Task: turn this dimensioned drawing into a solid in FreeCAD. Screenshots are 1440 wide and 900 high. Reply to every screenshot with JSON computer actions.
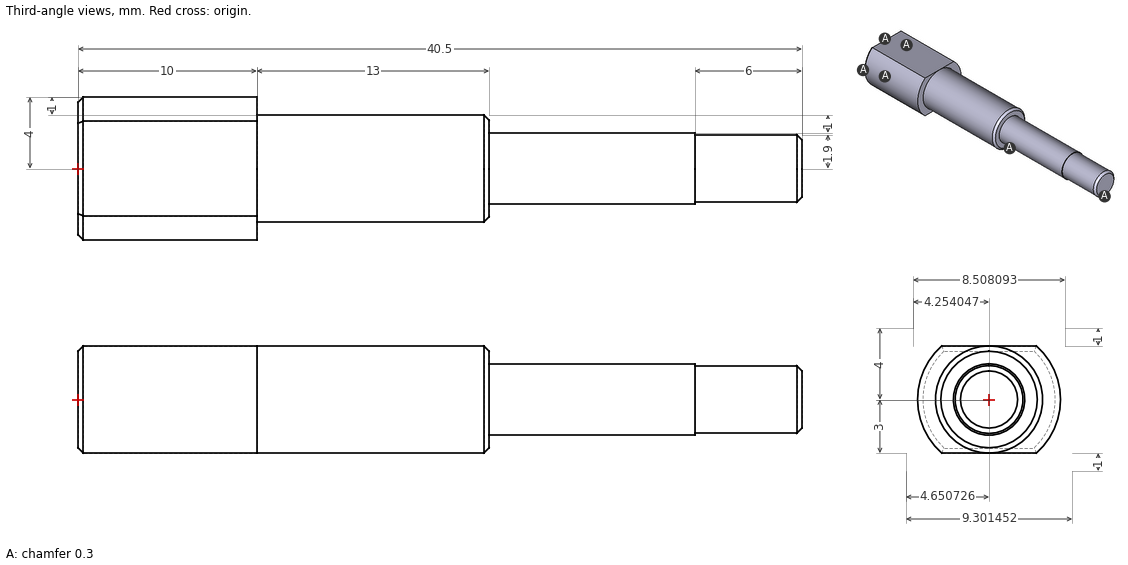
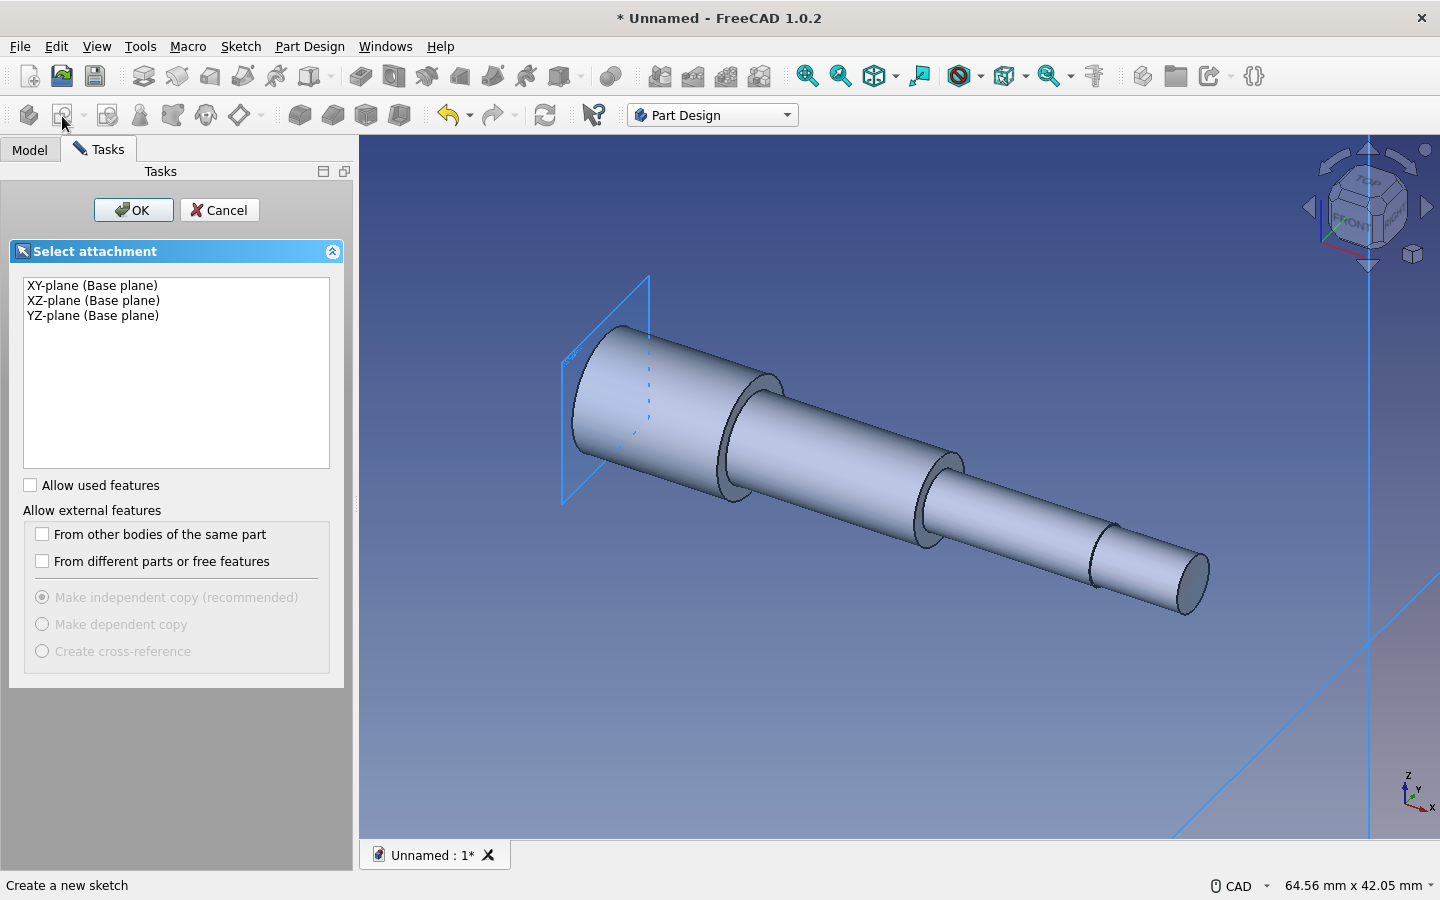
{"action": "left_click", "coordinate": [84, 316]}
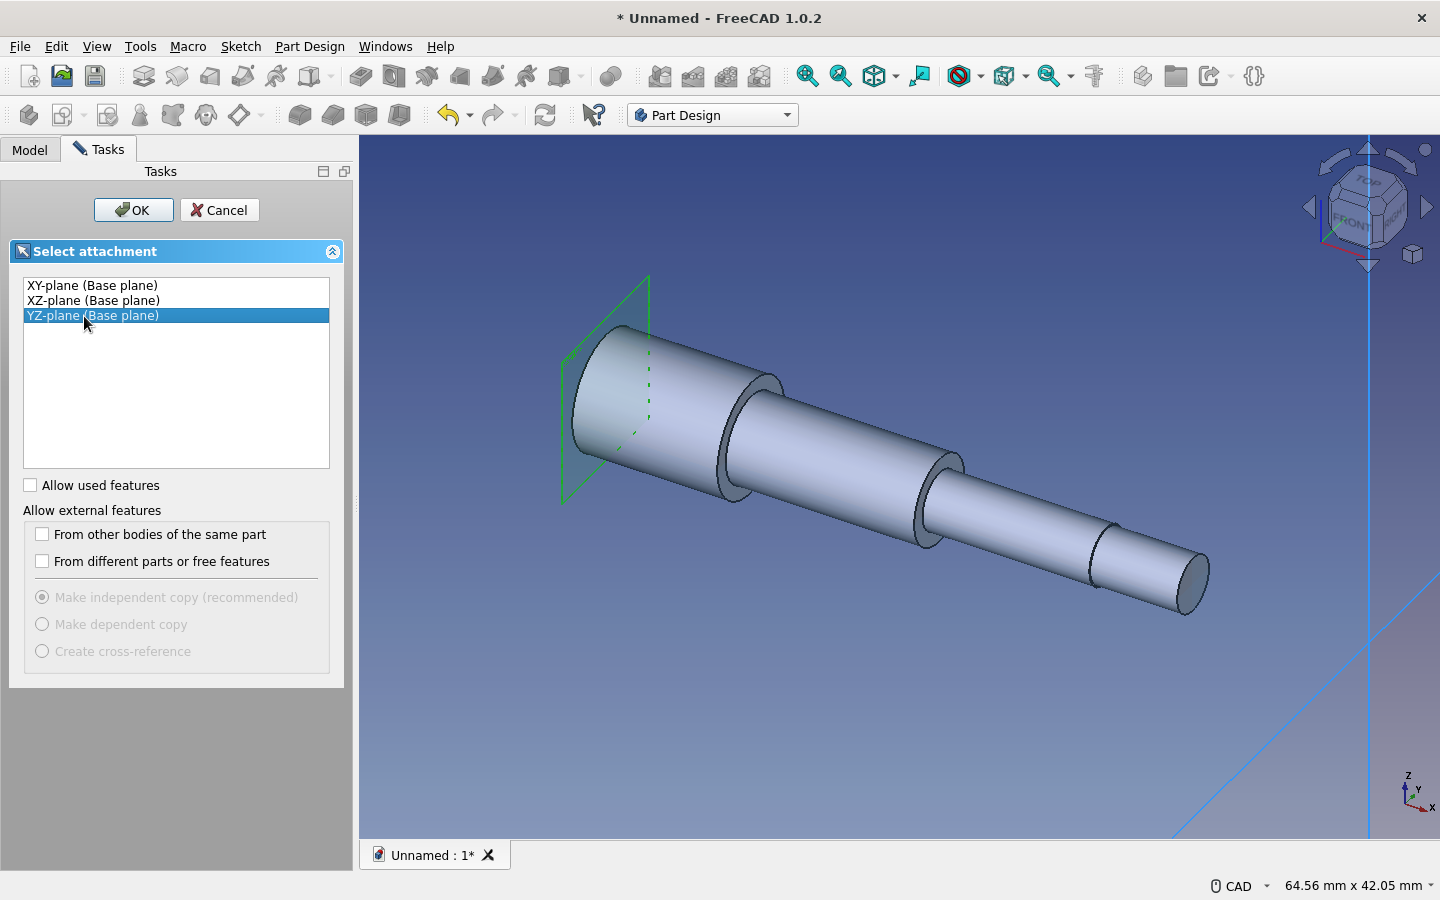
{"action": "left_click", "coordinate": [134, 210]}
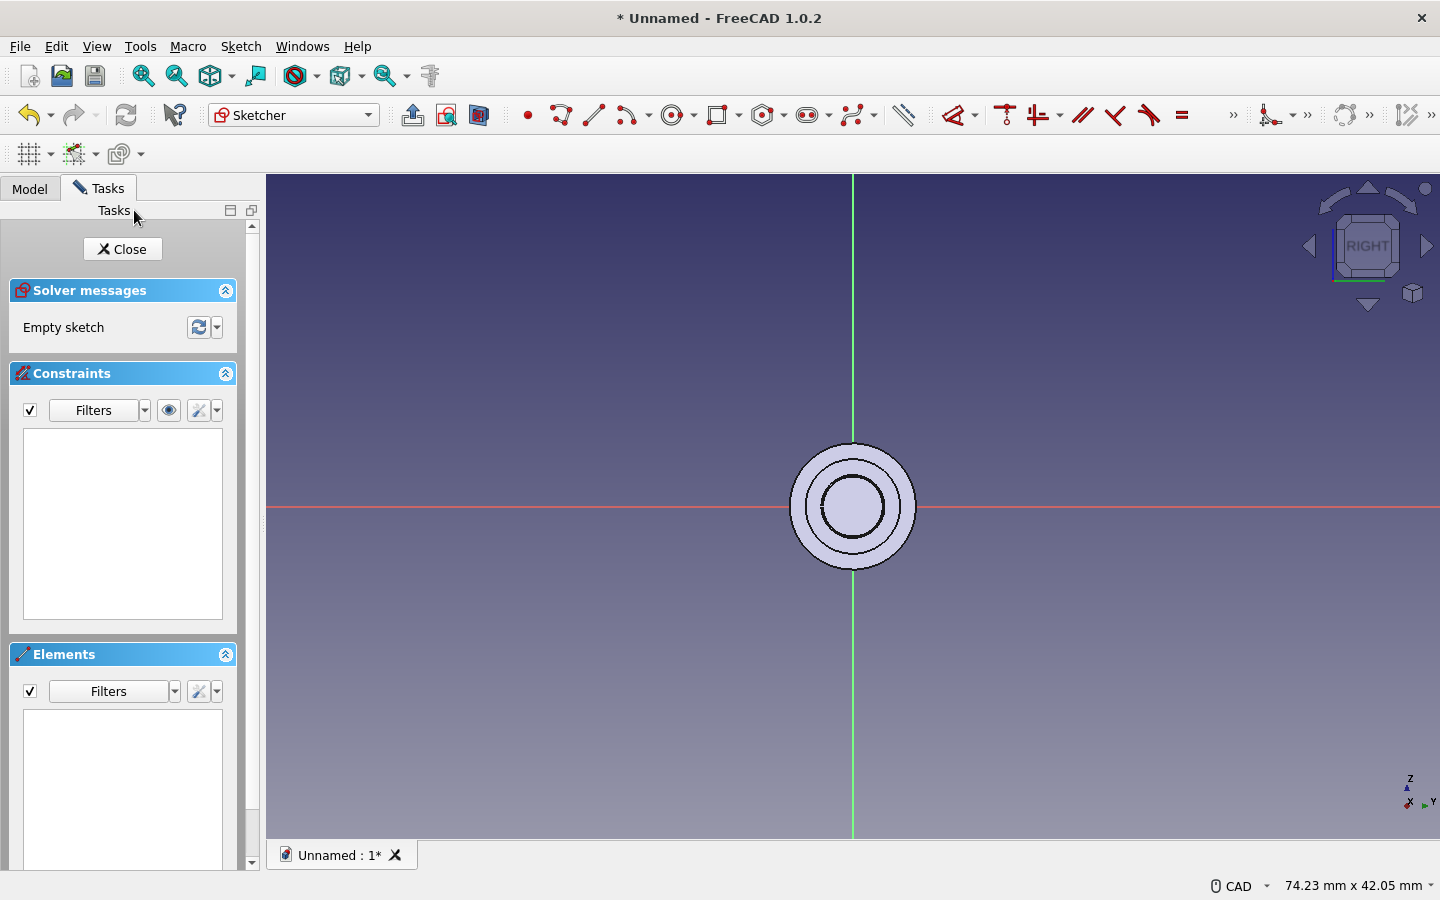
{"action": "left_click", "coordinate": [479, 116]}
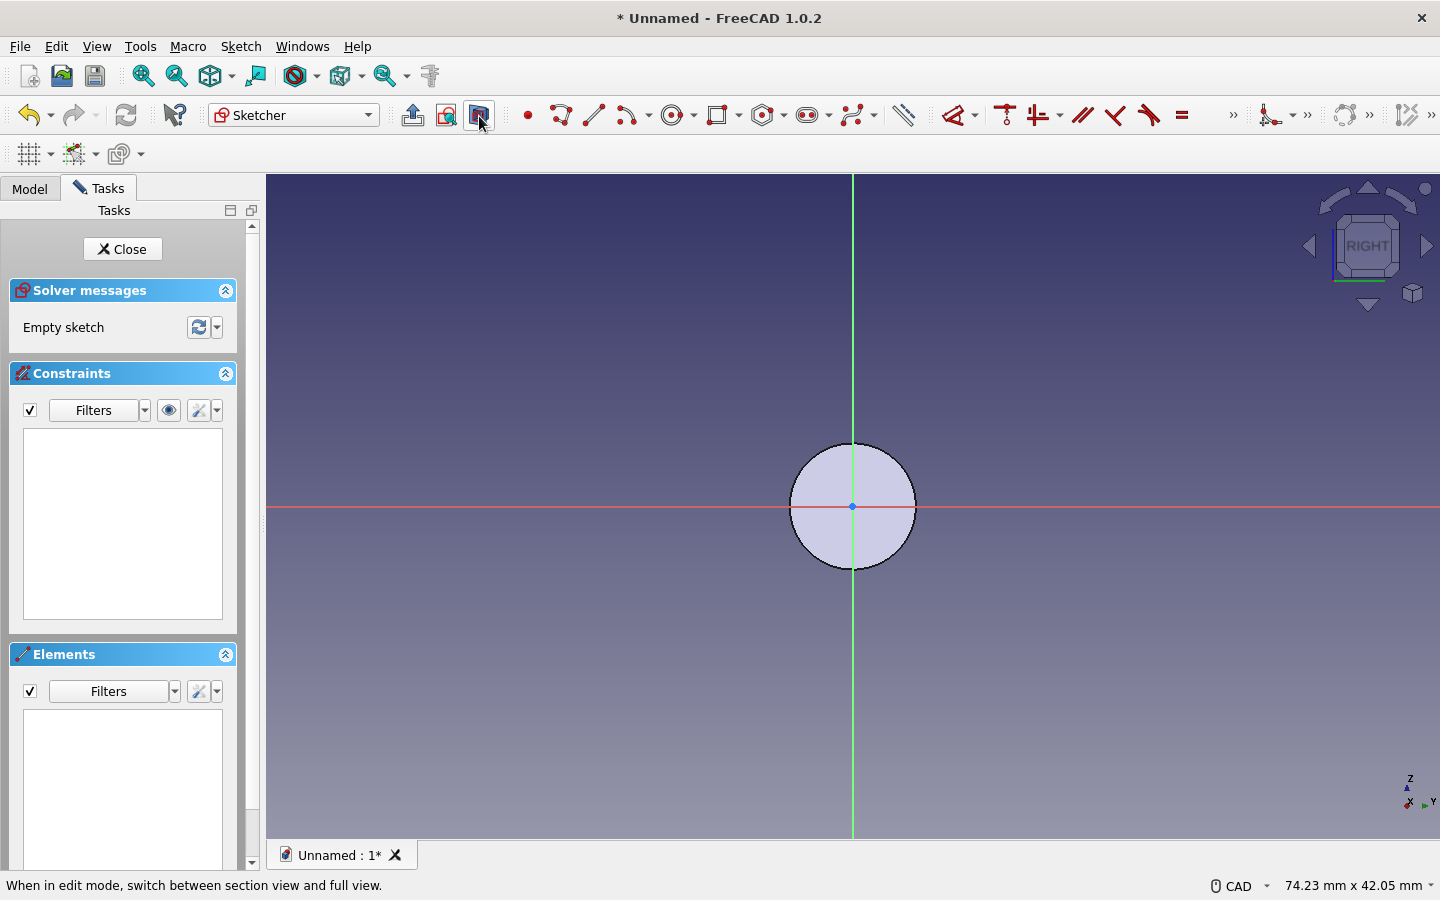
{"action": "scroll", "coordinate": [870, 546], "scroll_direction": "up", "scroll_amount": 8}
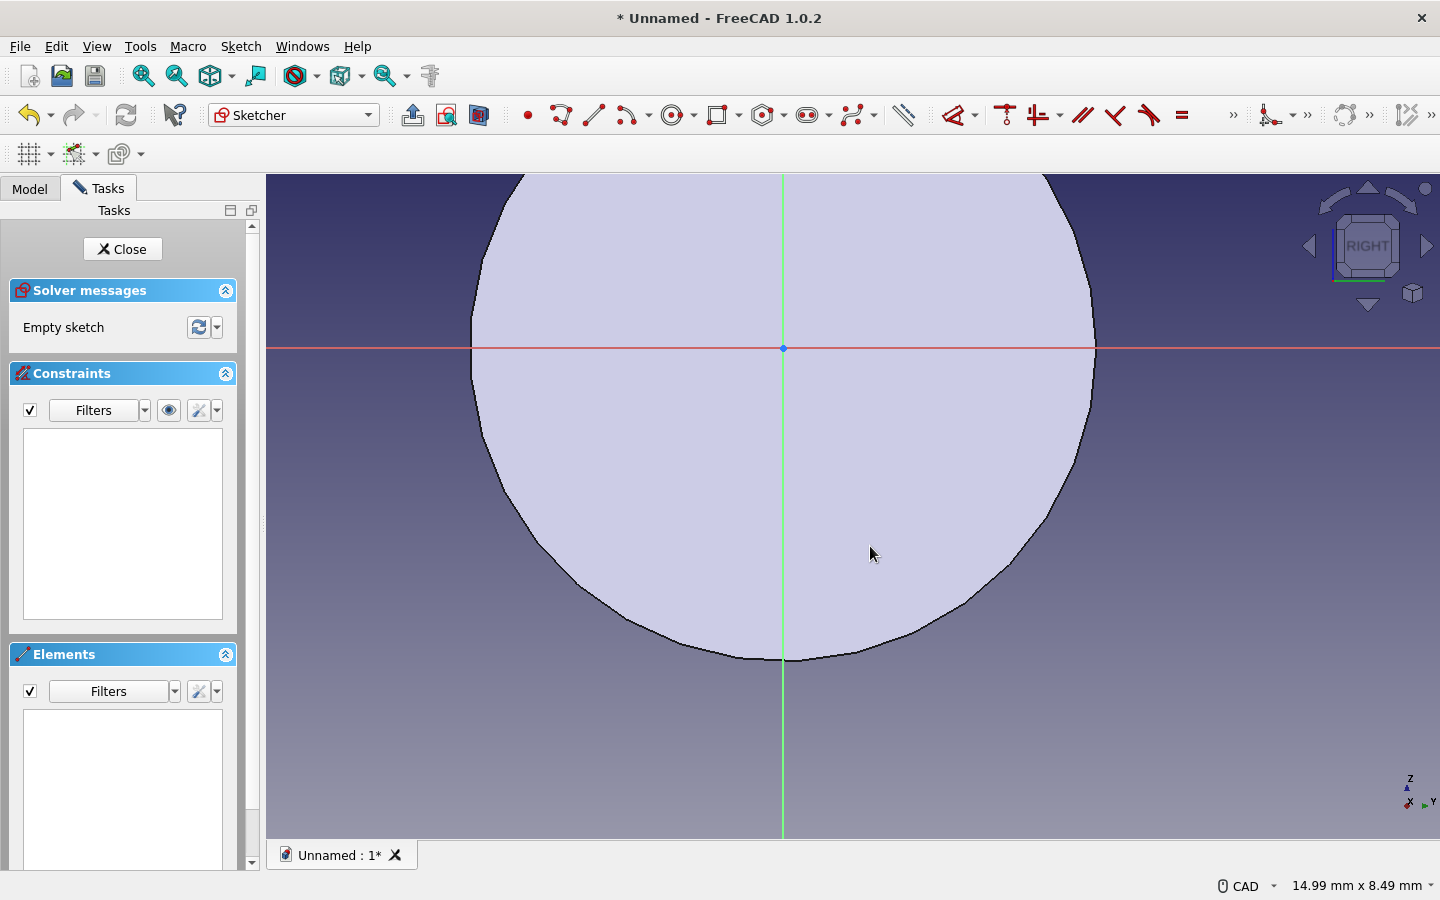
{"action": "left_click", "coordinate": [716, 116]}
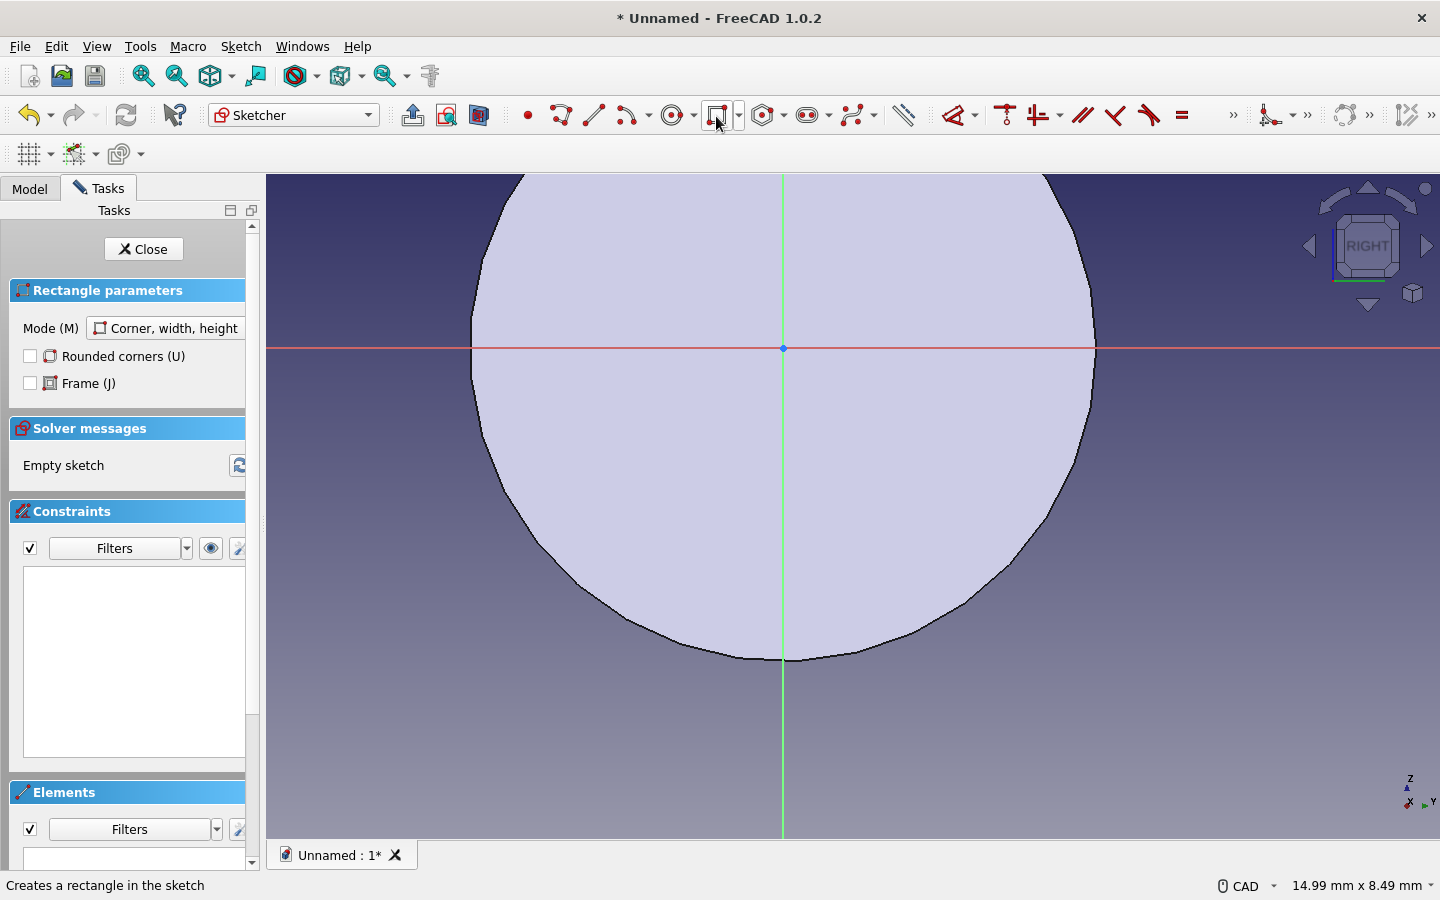
{"action": "left_click", "coordinate": [419, 583]}
{"action": "mouse_move", "coordinate": [1147, 661]}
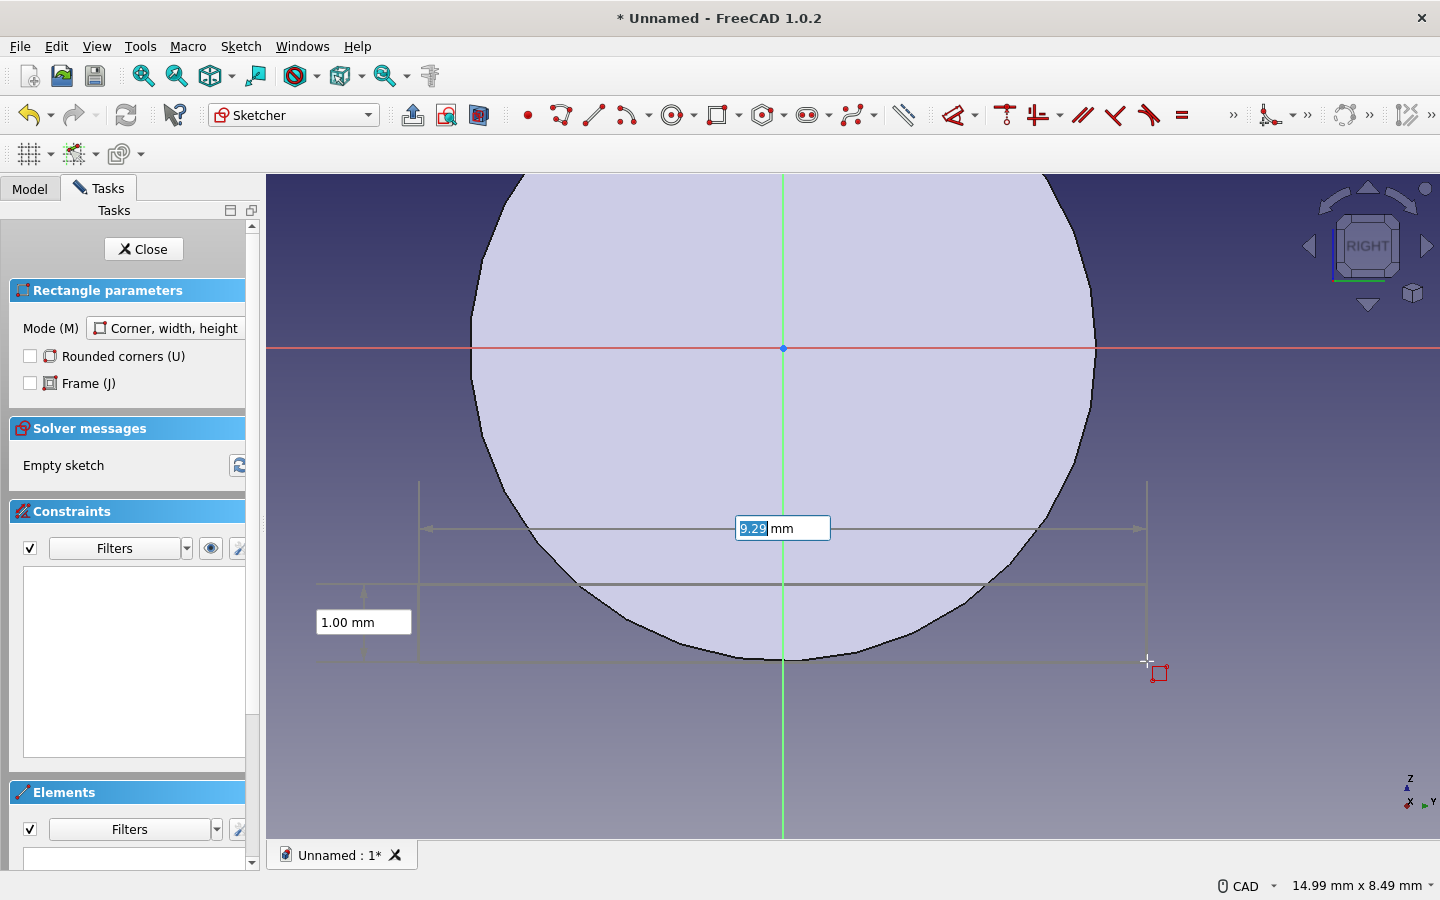
{"action": "type", "text": "9.301452"}
{"action": "key", "text": "Tab"}
{"action": "type", "text": "1"}
{"action": "key", "text": "Return"}
{"action": "key", "text": "Escape"}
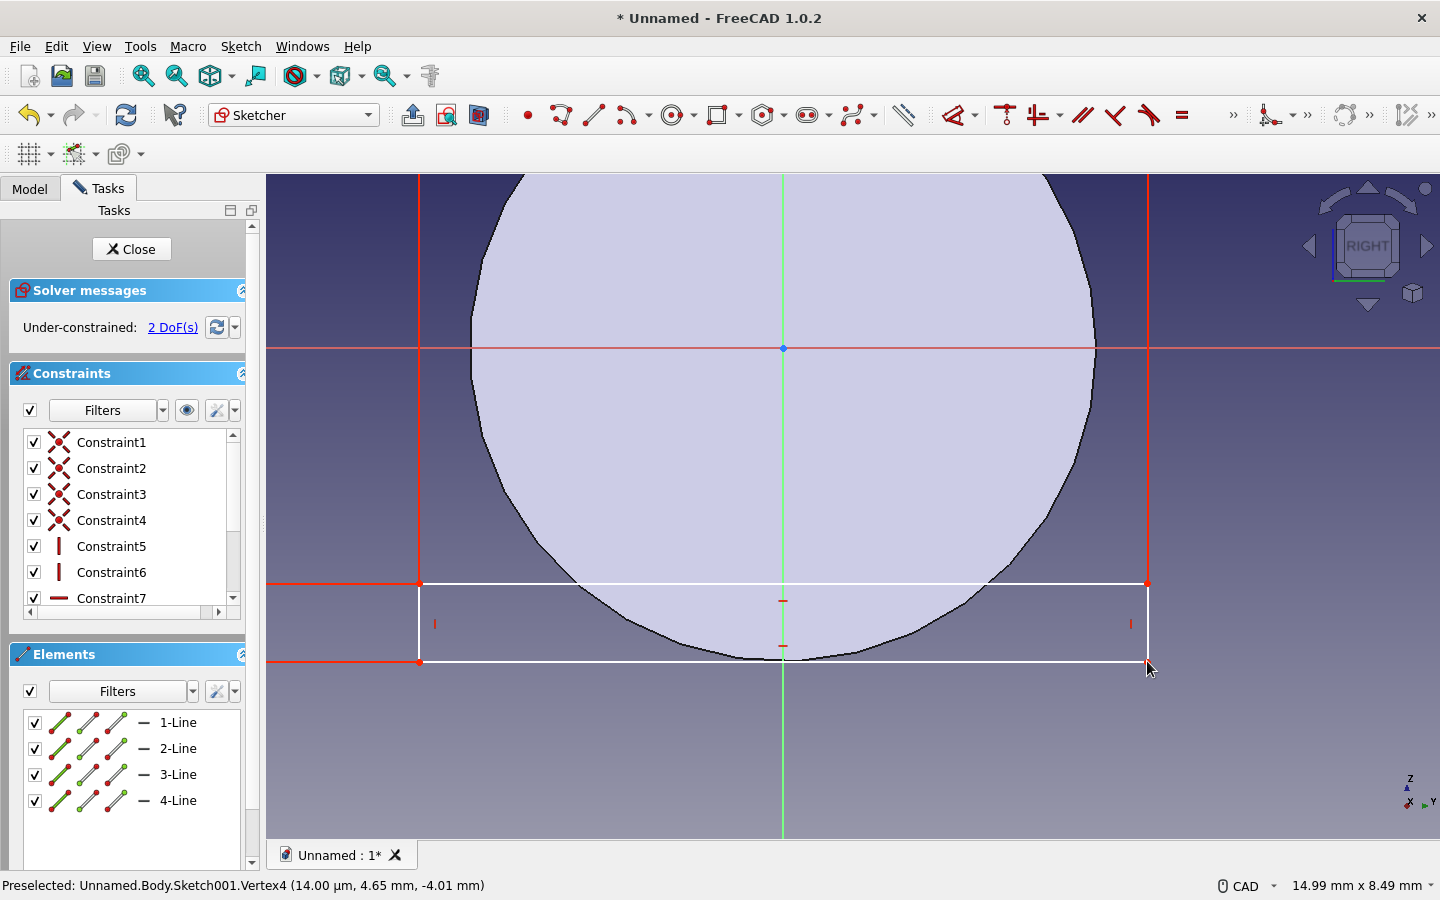
{"action": "key", "text": "d"}